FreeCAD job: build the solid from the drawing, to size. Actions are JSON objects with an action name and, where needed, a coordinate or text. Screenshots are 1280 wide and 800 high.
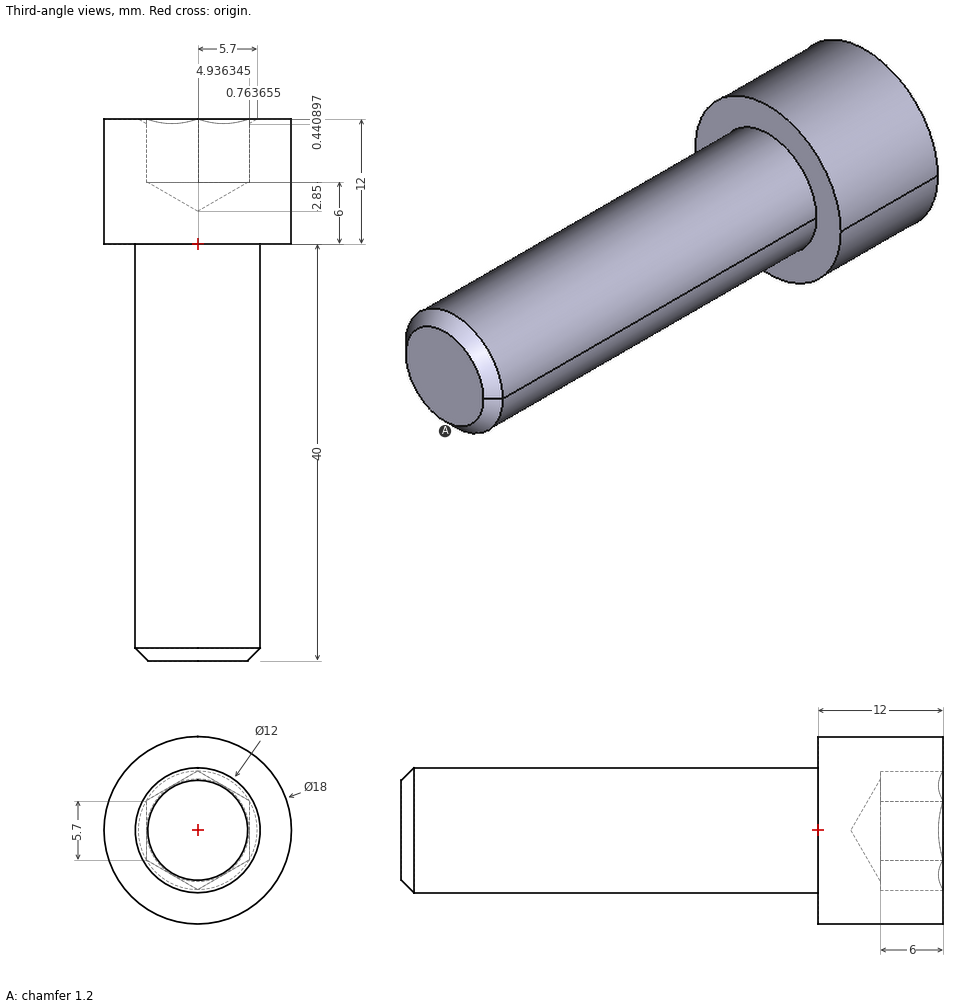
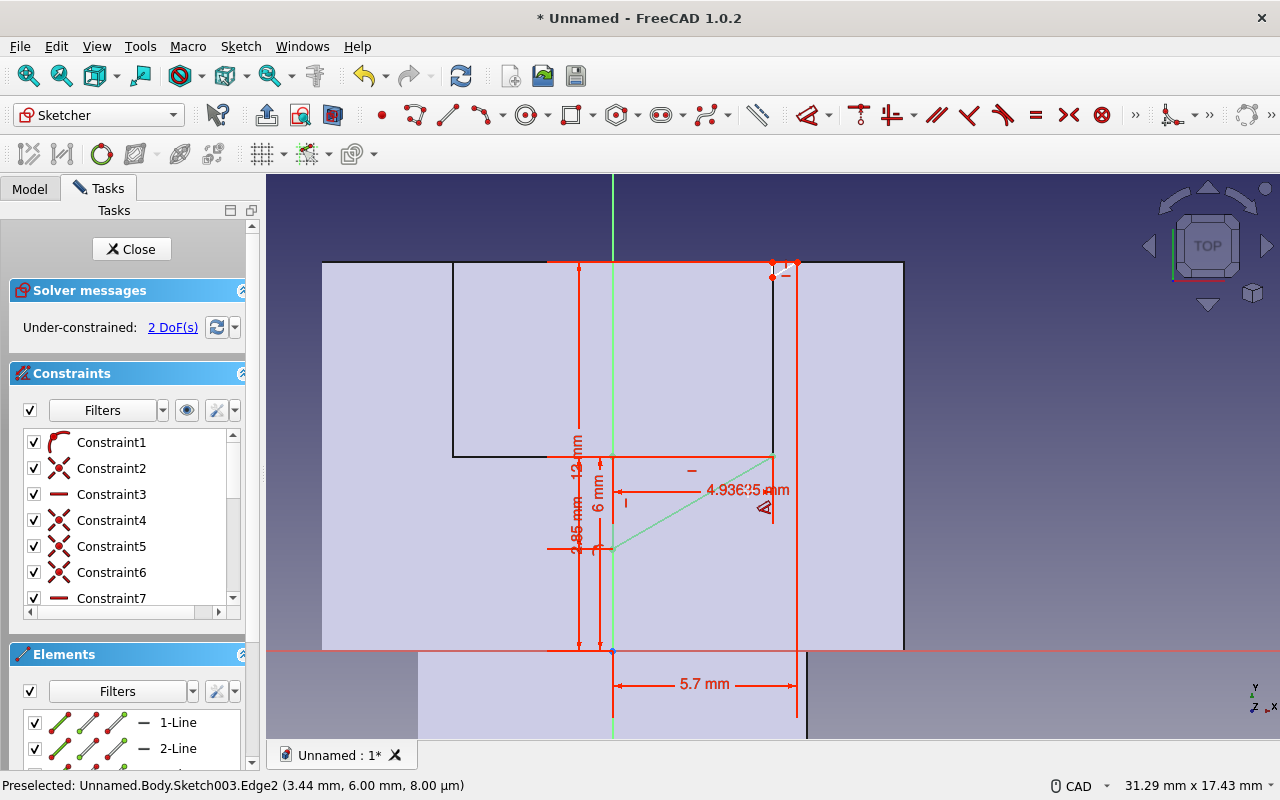
{"action": "scroll", "coordinate": [782, 262], "scroll_direction": "up", "scroll_amount": 3}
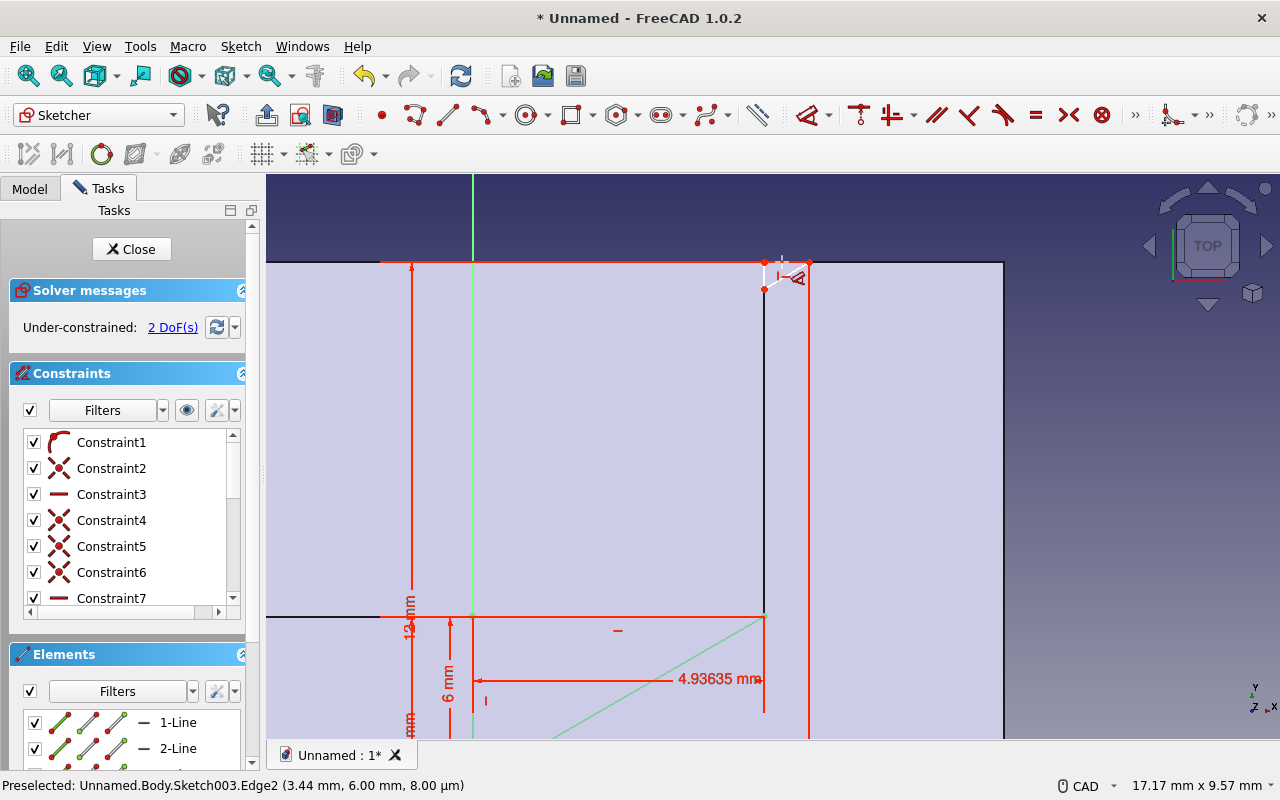
{"action": "left_click", "coordinate": [782, 262]}
{"action": "left_click", "coordinate": [787, 228]}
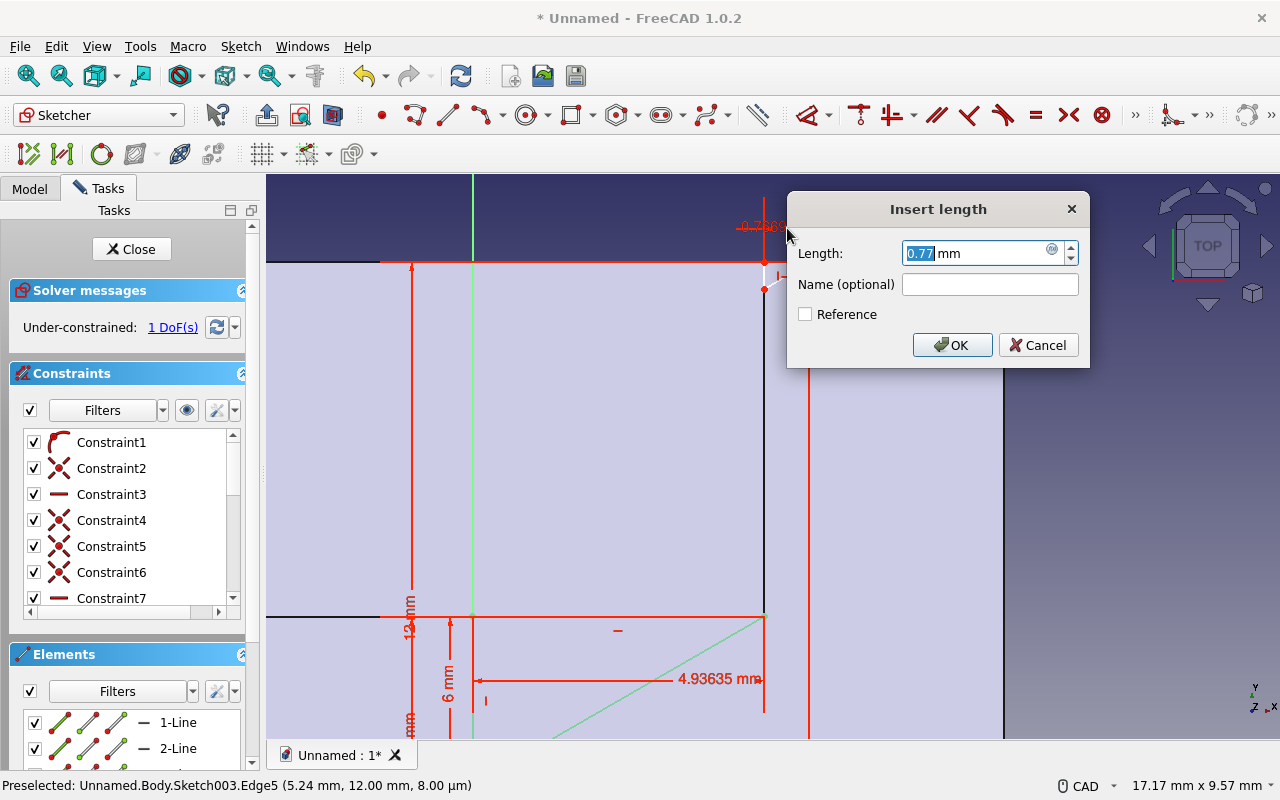
{"action": "type", "text": "0.763655"}
{"action": "key", "text": "Return"}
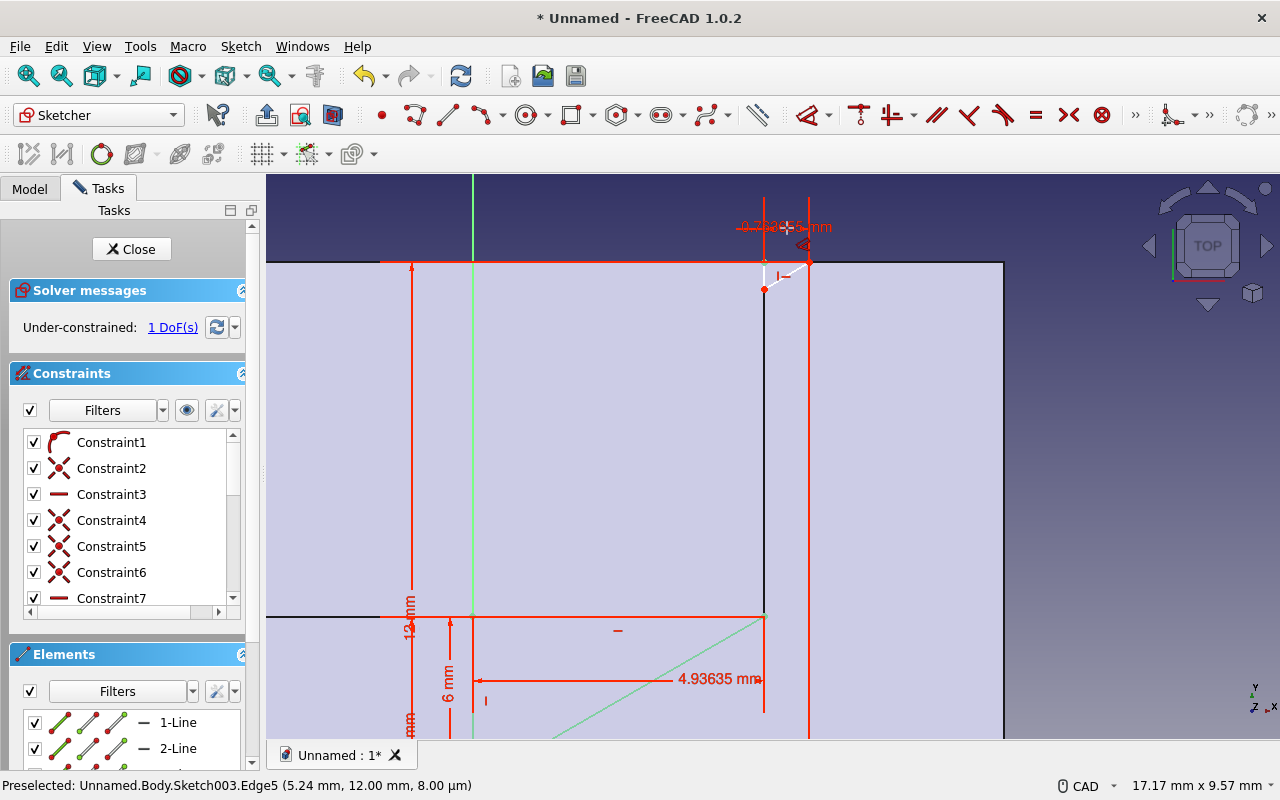
{"action": "scroll", "coordinate": [764, 273], "scroll_direction": "up", "scroll_amount": 3}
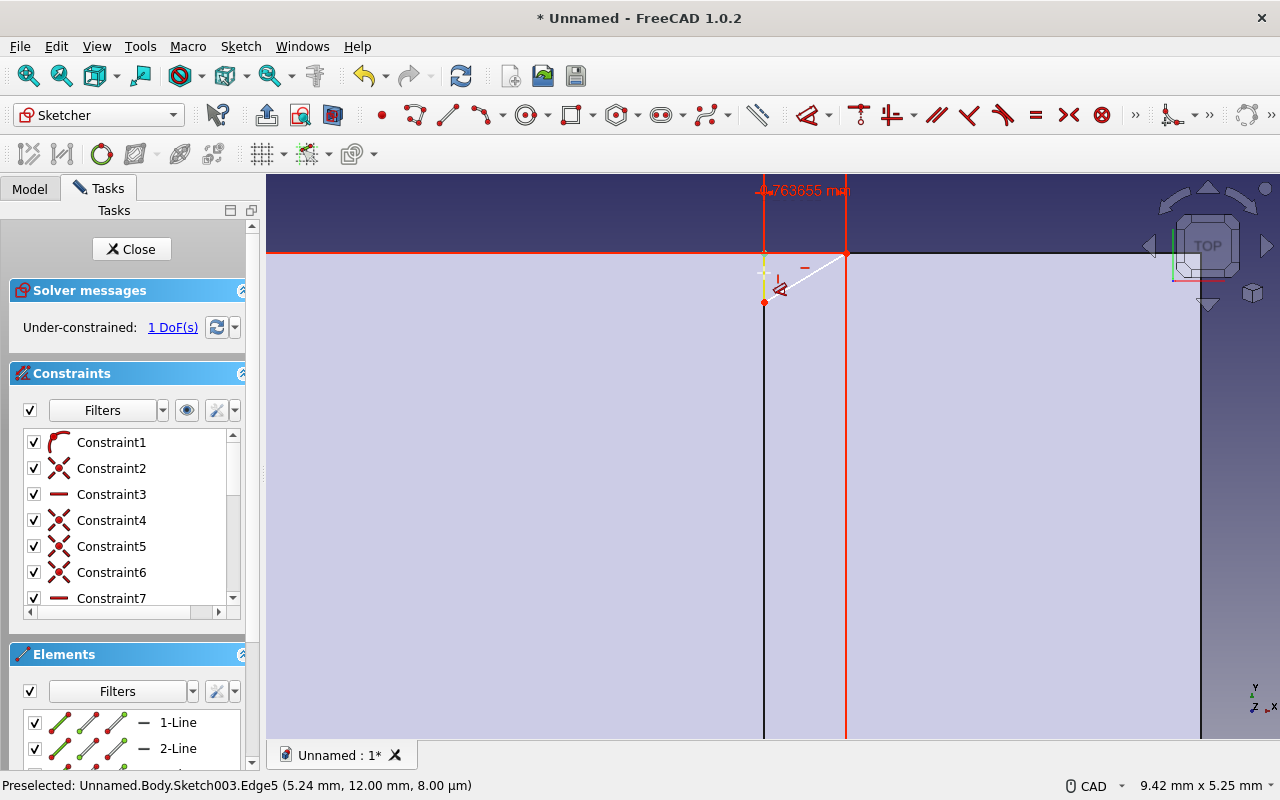
{"action": "left_click", "coordinate": [764, 273]}
{"action": "left_click", "coordinate": [798, 267]}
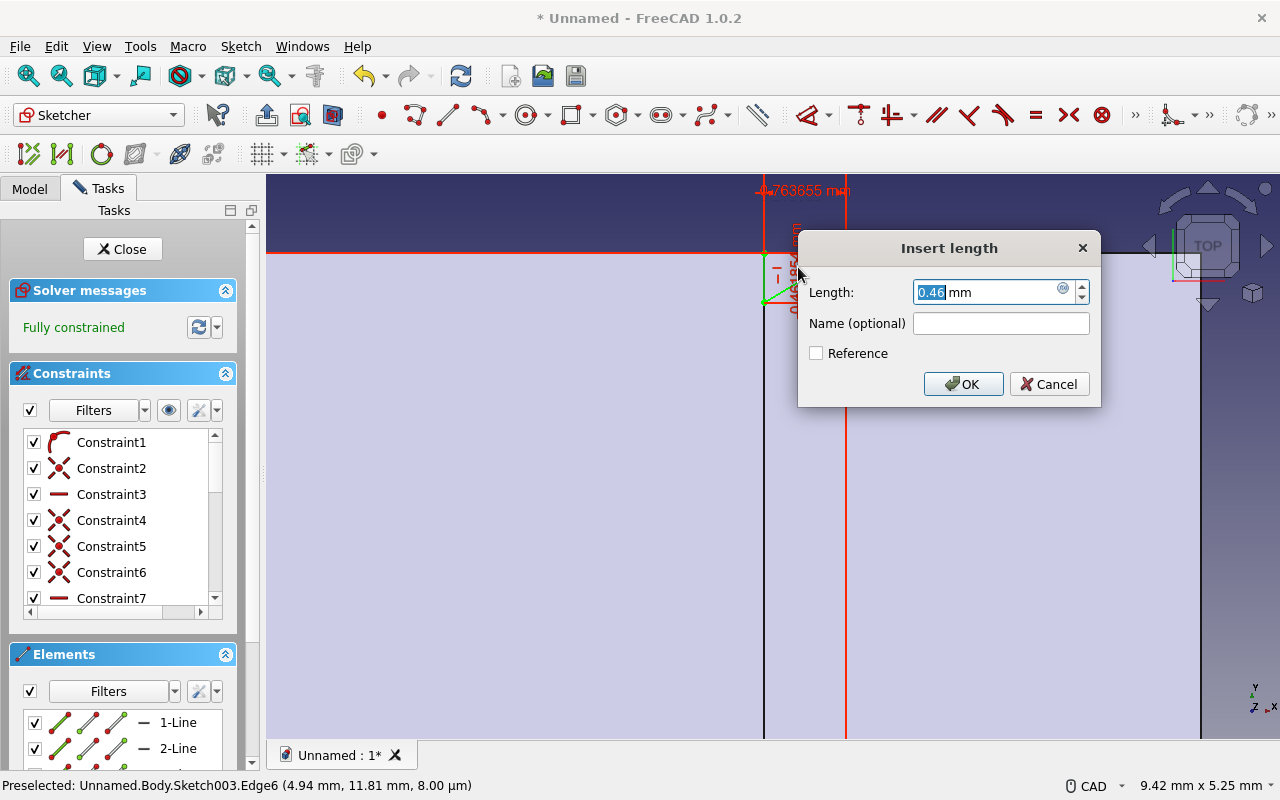
{"action": "type", "text": "0.440897"}
{"action": "key", "text": "Return"}
{"action": "key", "text": "Escape"}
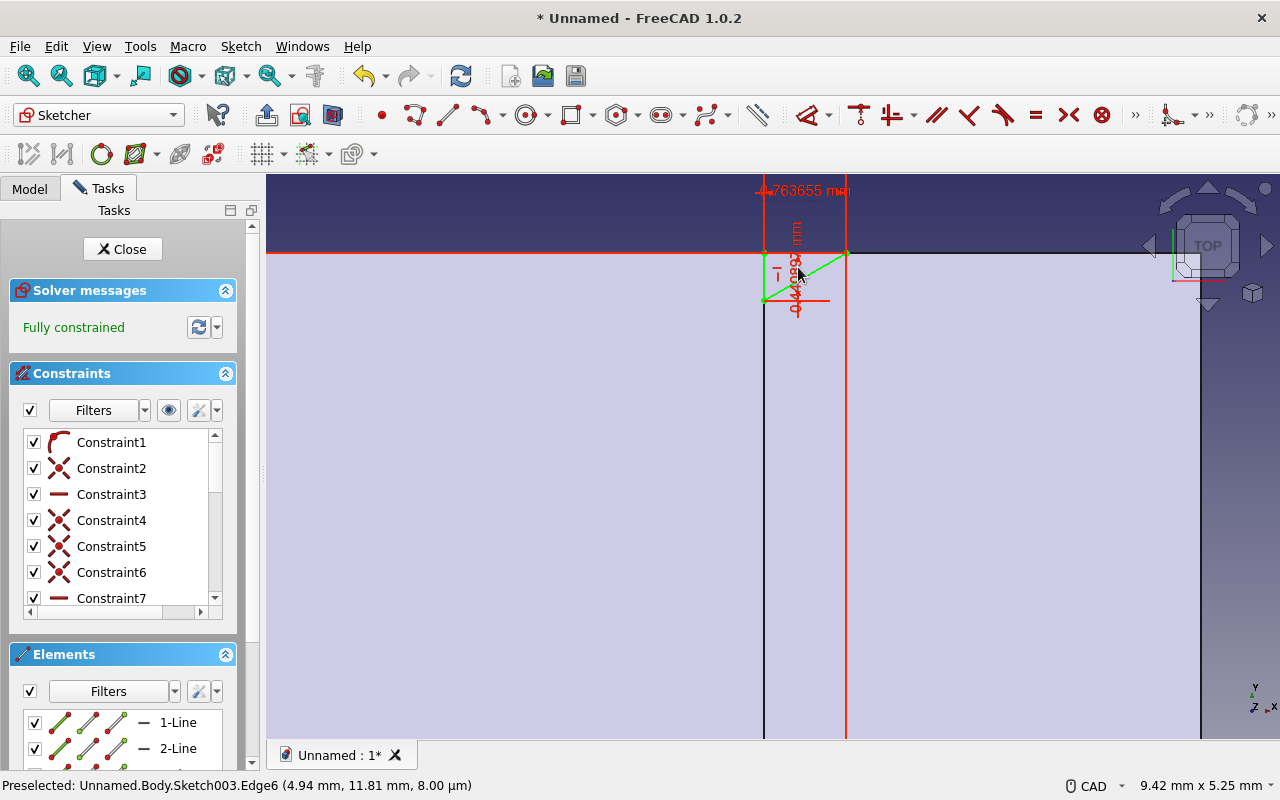
{"action": "left_click", "coordinate": [123, 249]}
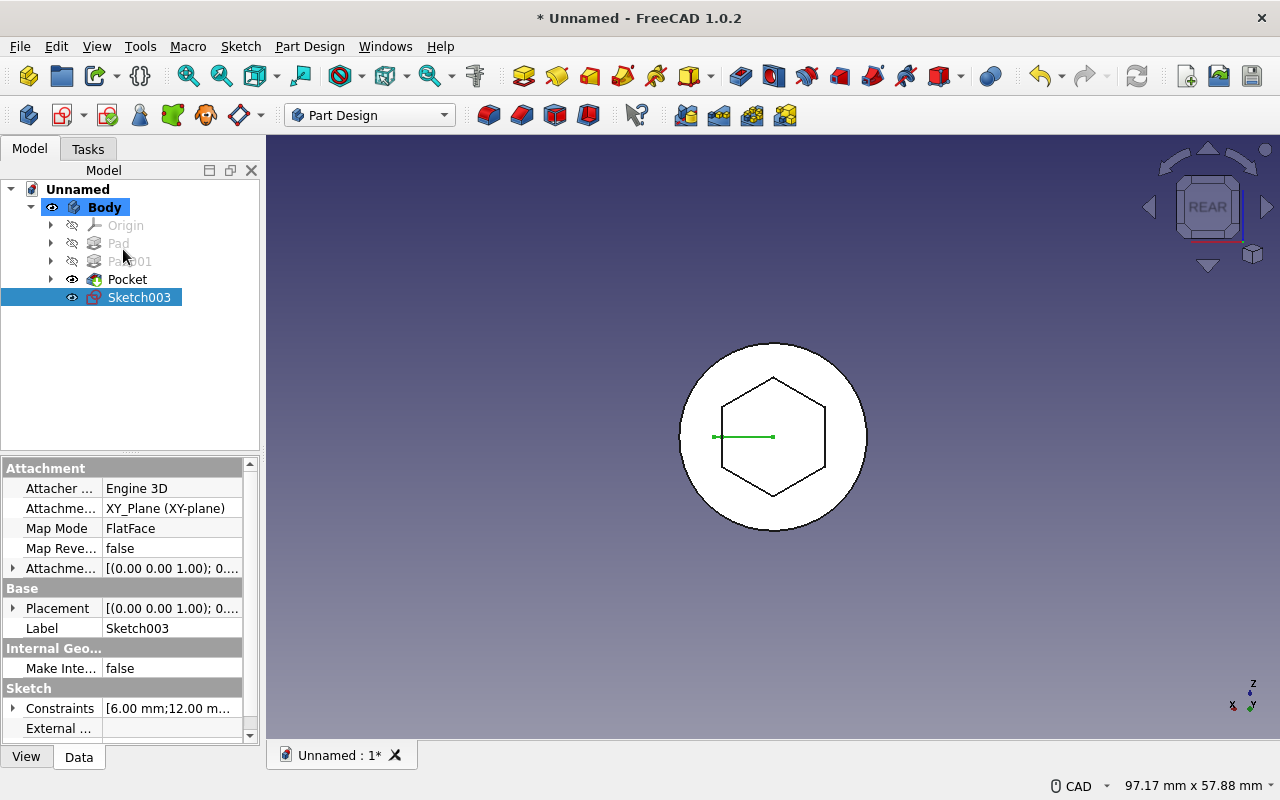
{"action": "left_click", "coordinate": [807, 76]}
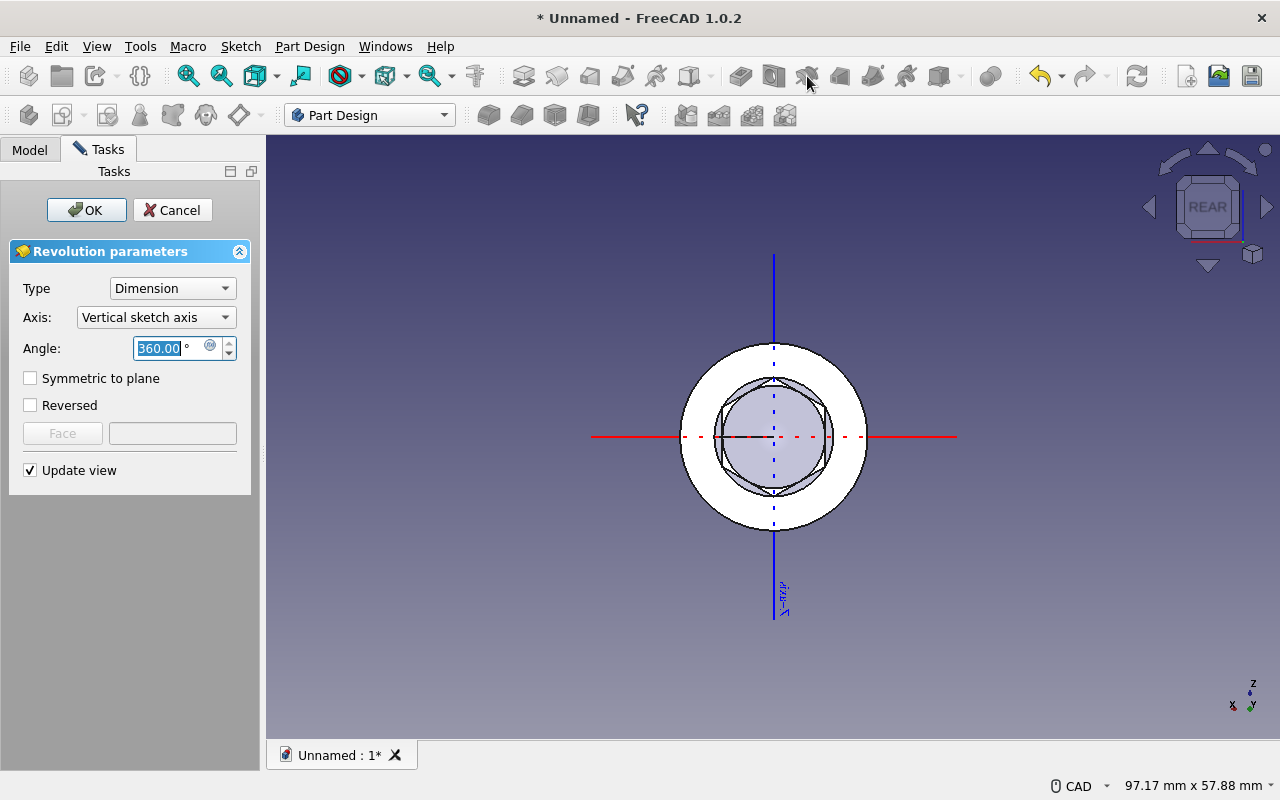
{"action": "left_click", "coordinate": [87, 210]}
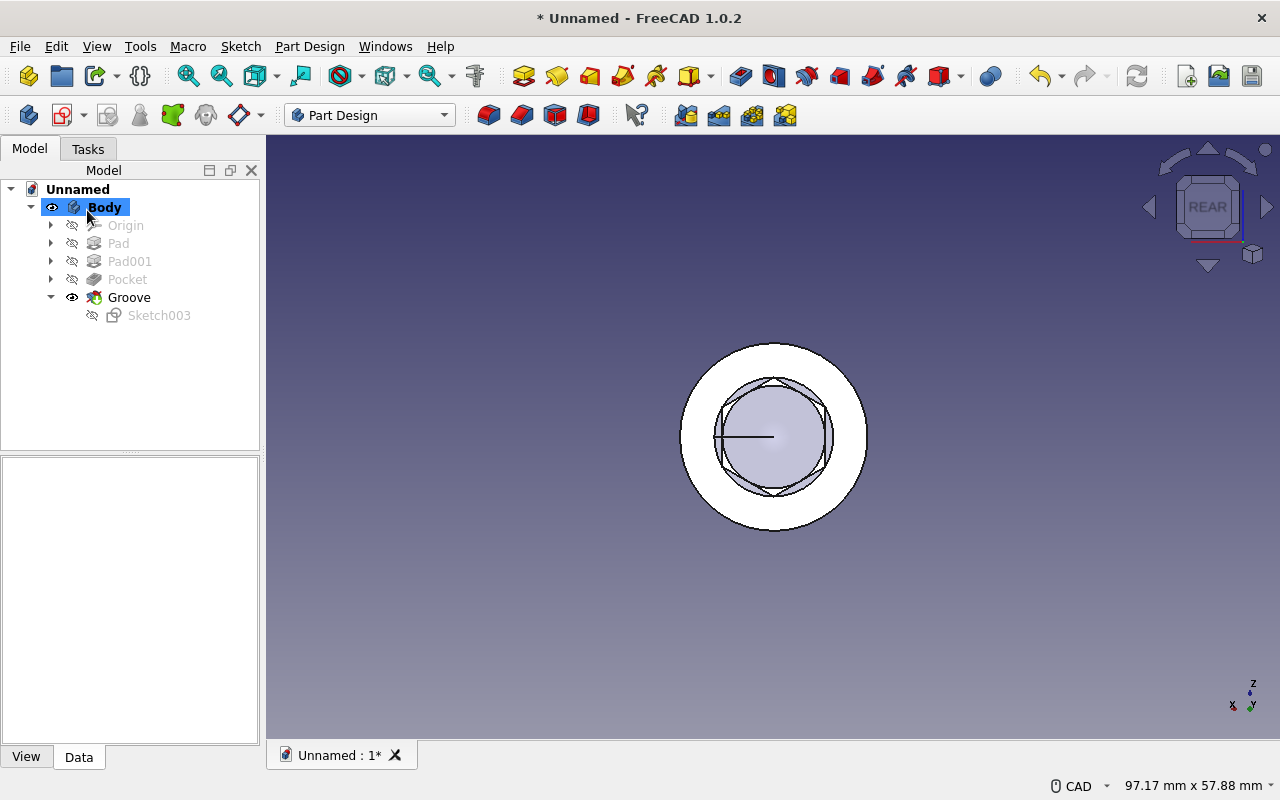
{"action": "left_click", "coordinate": [189, 76]}